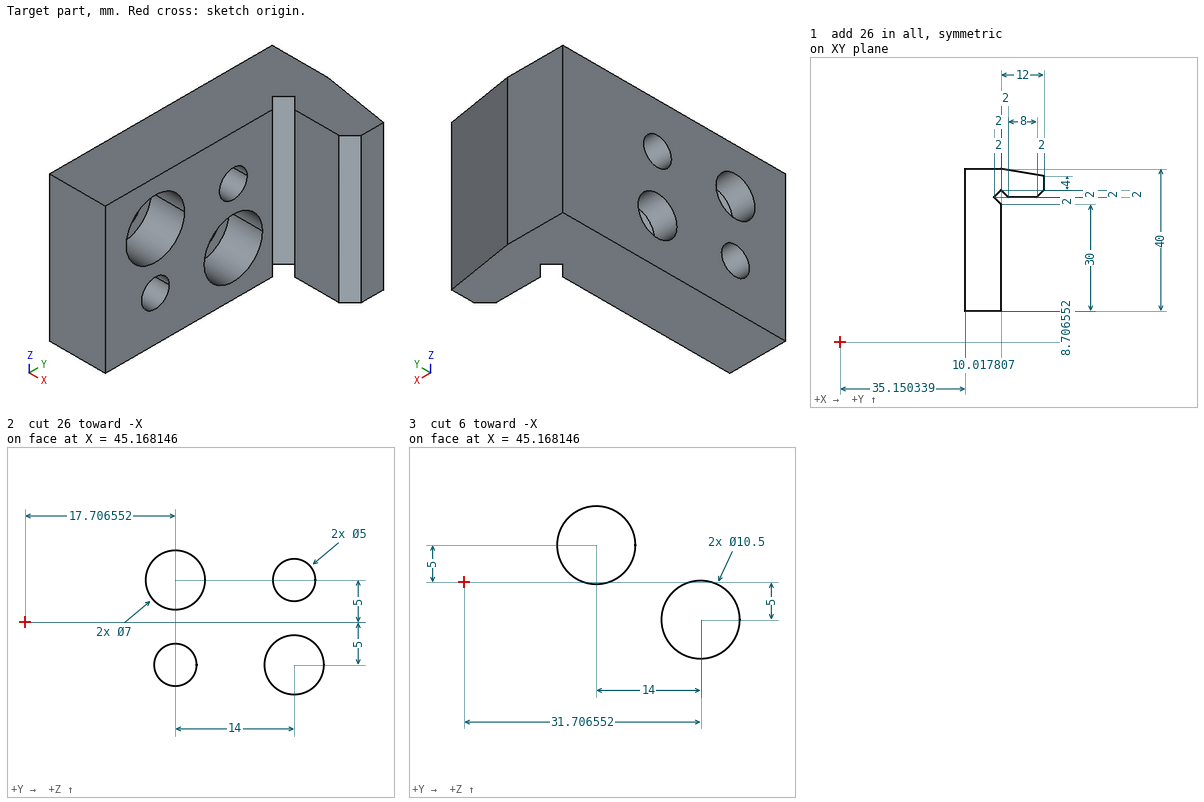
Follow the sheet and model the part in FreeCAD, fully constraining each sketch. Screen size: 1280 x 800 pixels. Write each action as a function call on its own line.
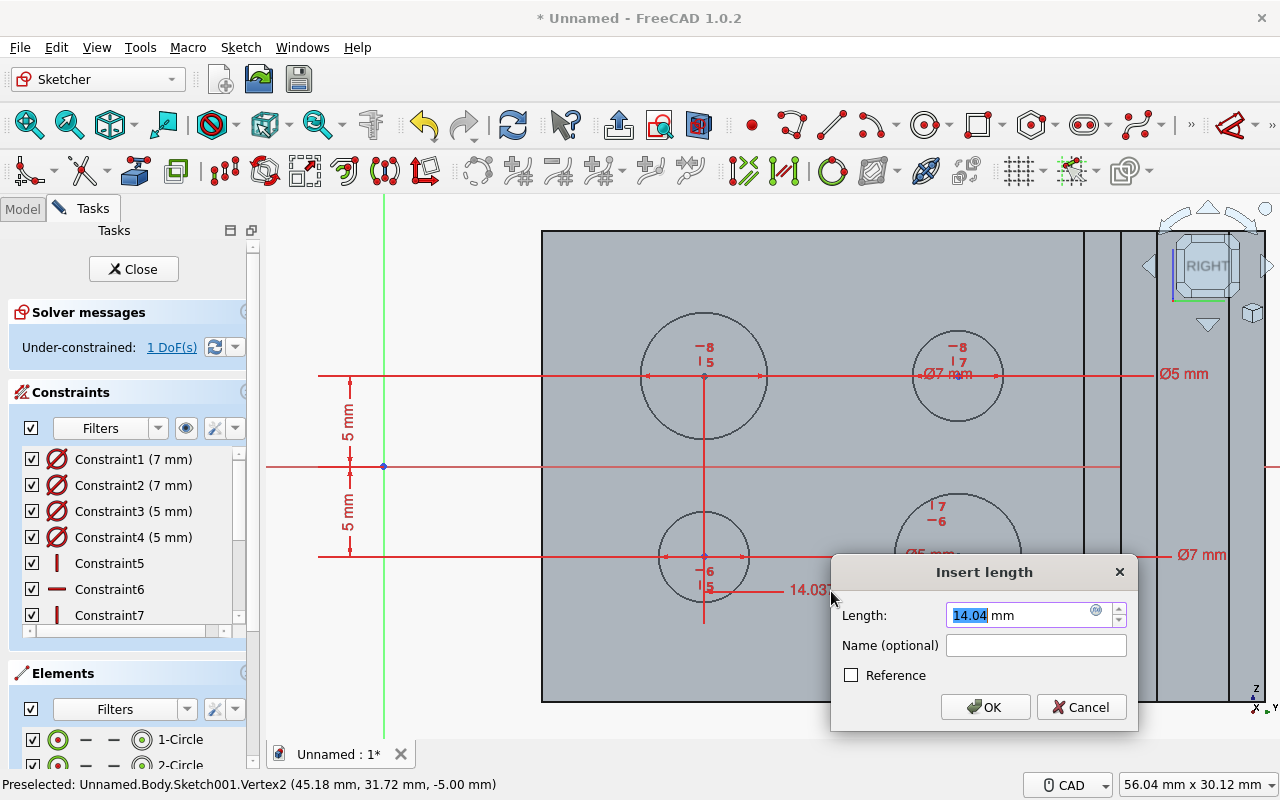
text(14)
key(Return)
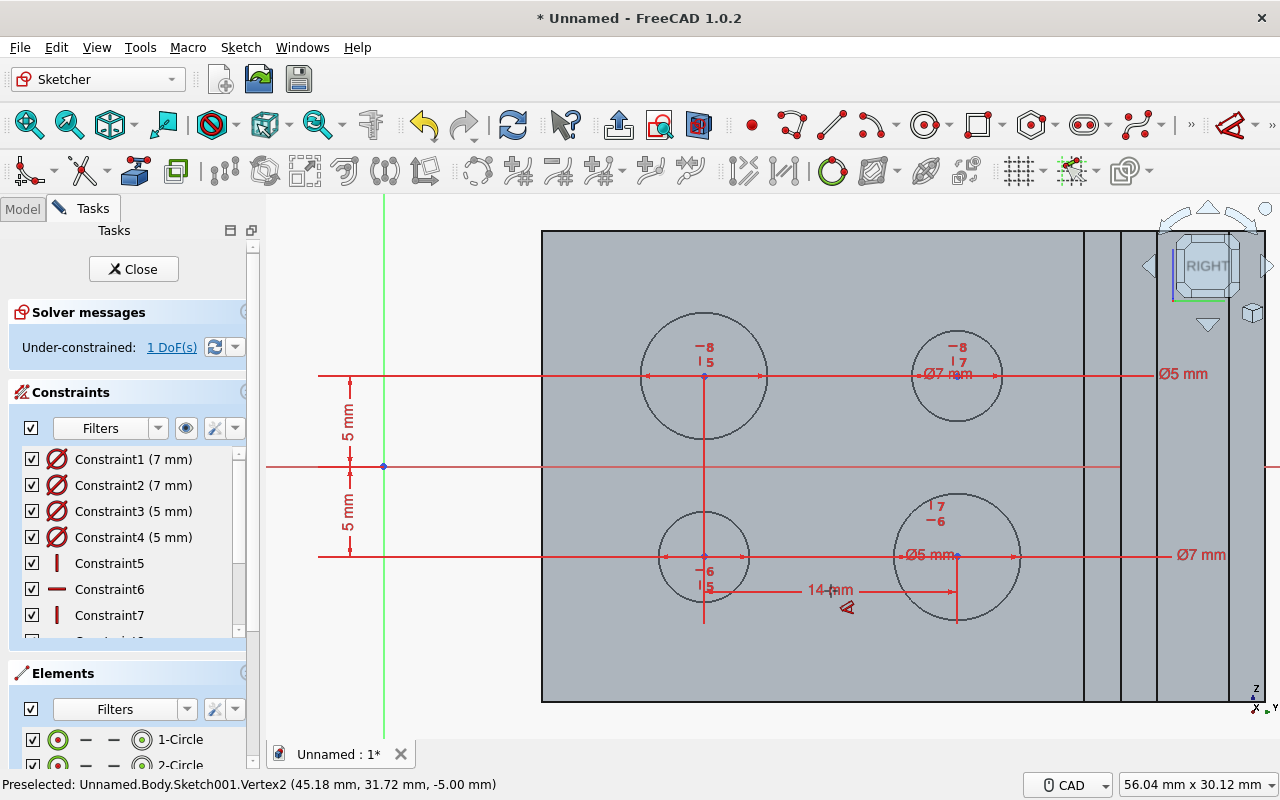
click(704, 376)
click(544, 342)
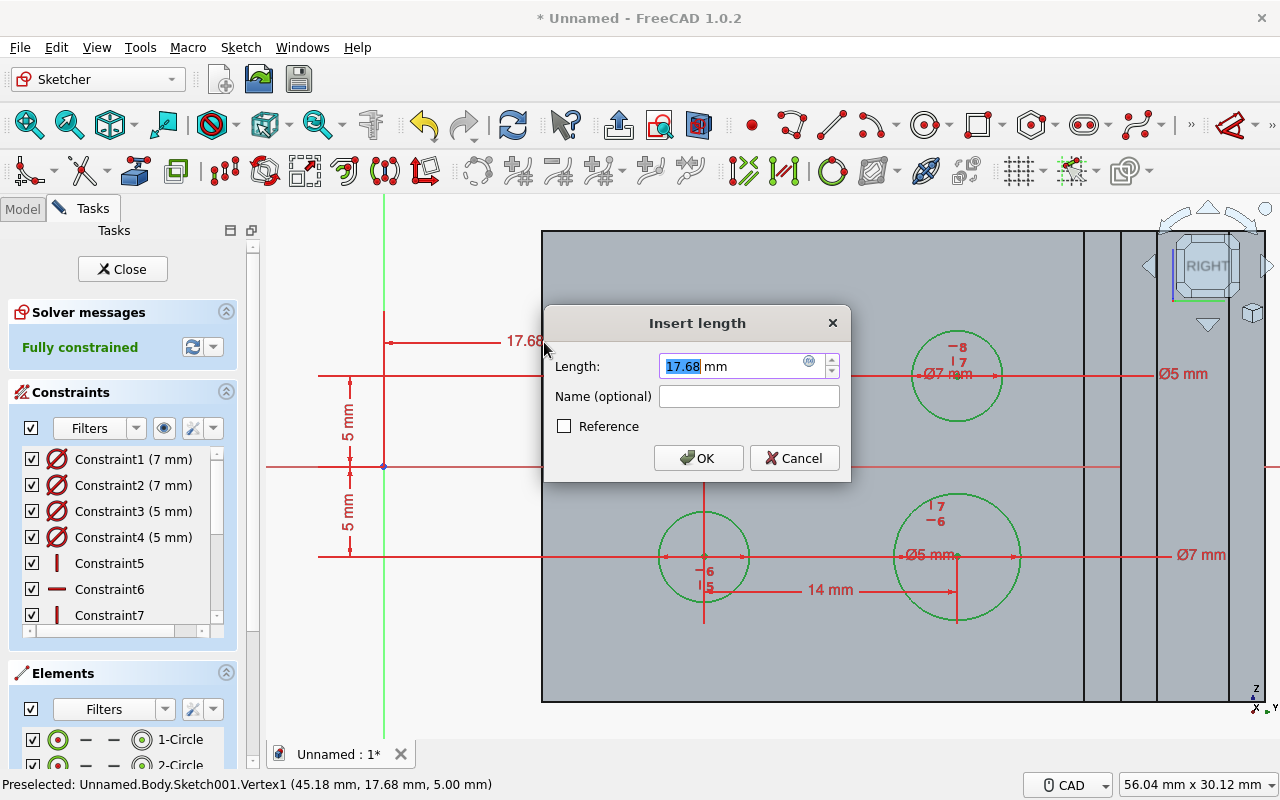
text(17.706552)
key(Return)
key(Escape)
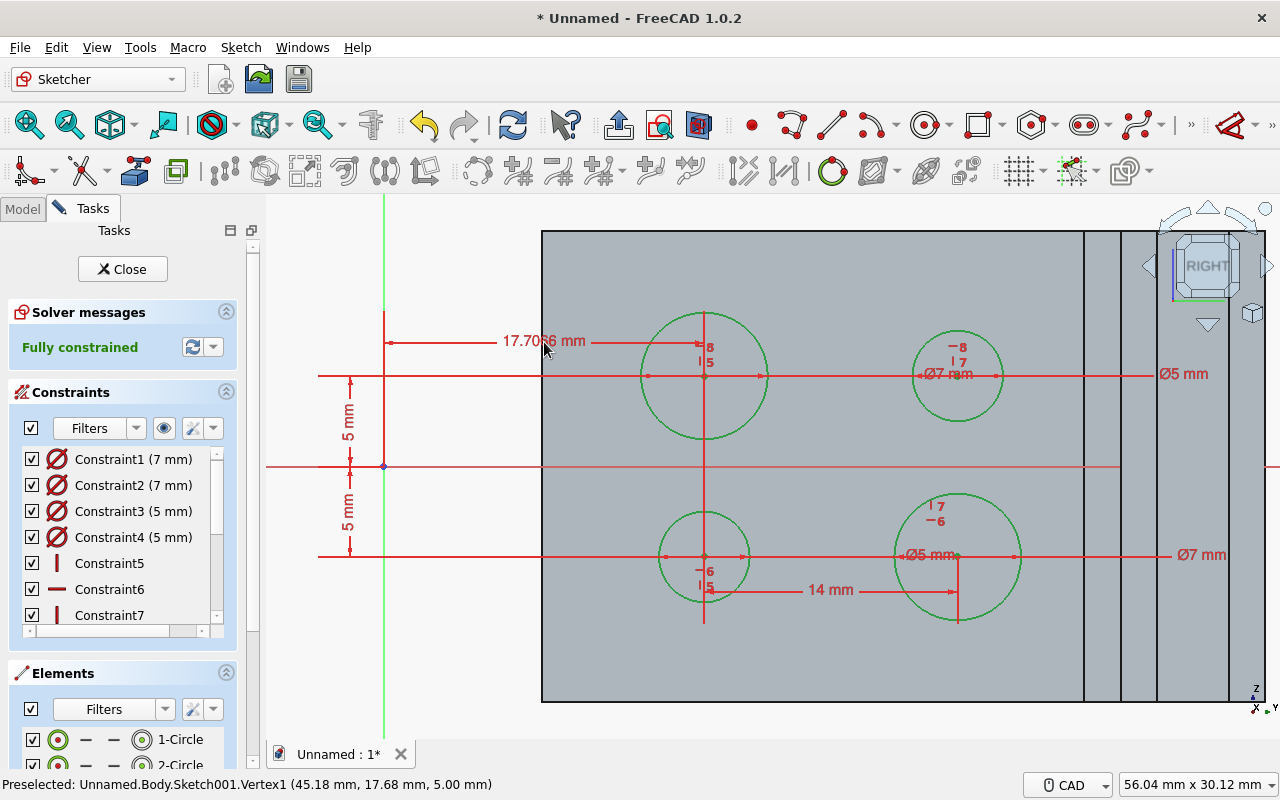
click(123, 269)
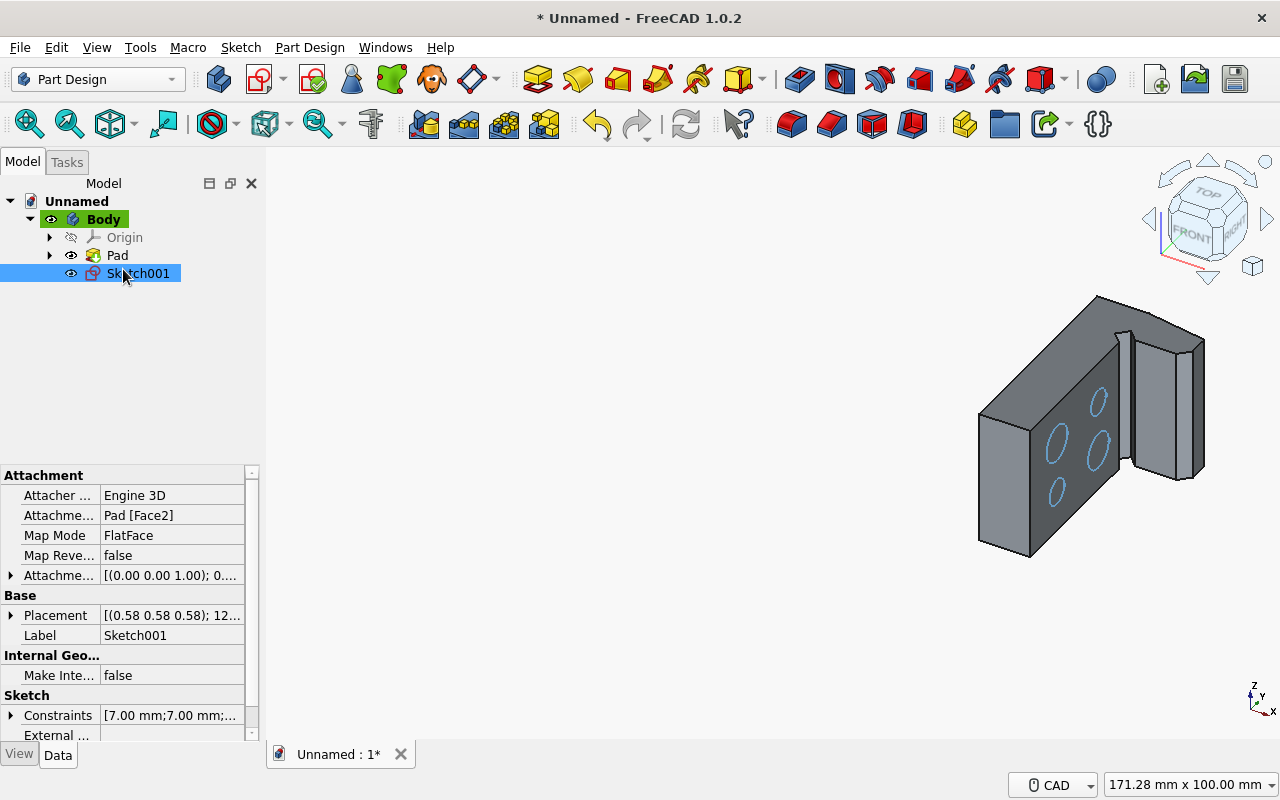
click(800, 80)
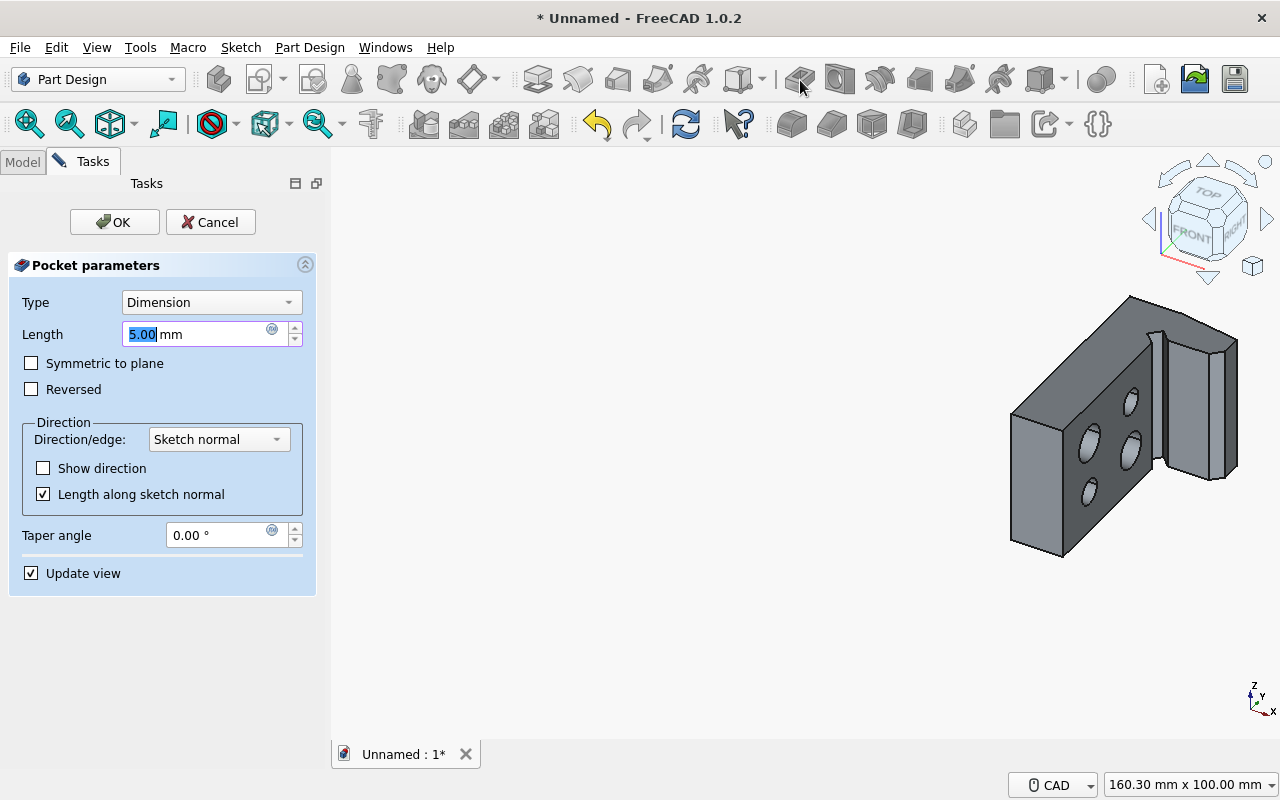
text(26)
key(Tab)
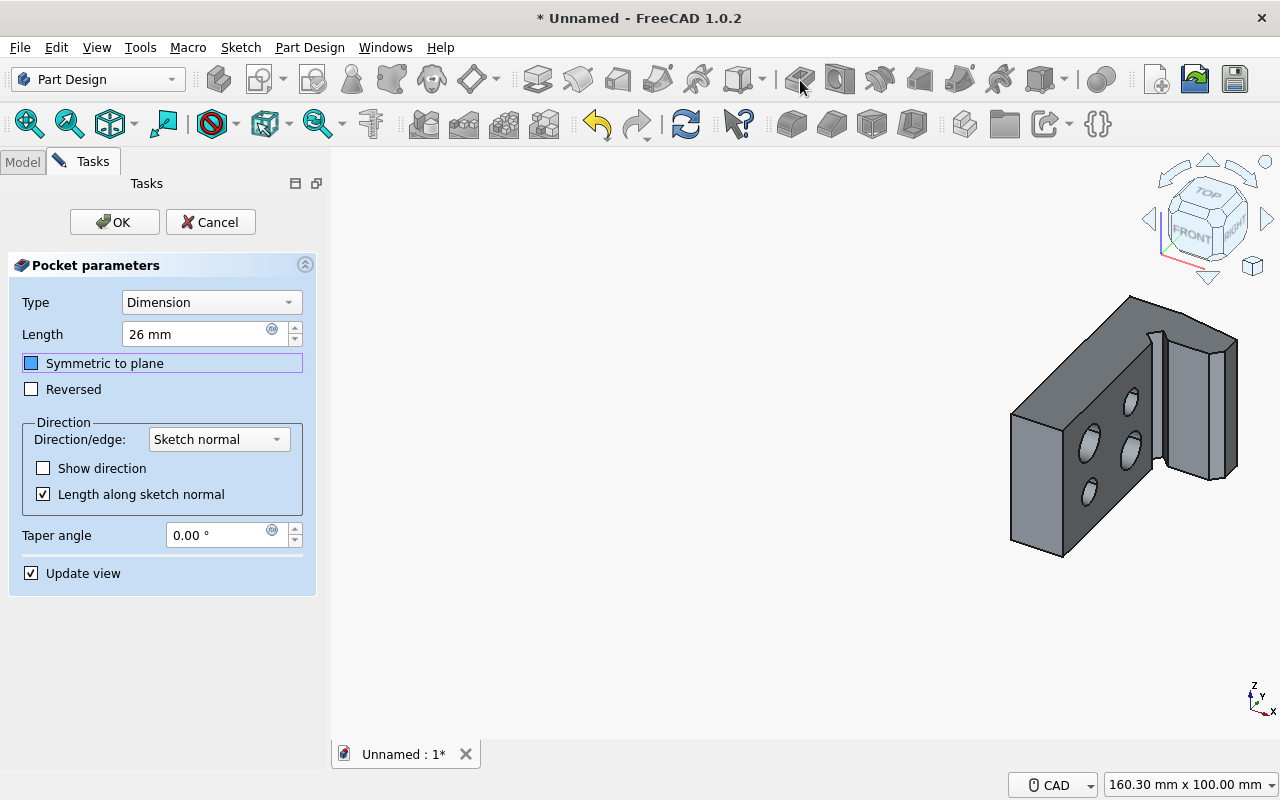
click(115, 222)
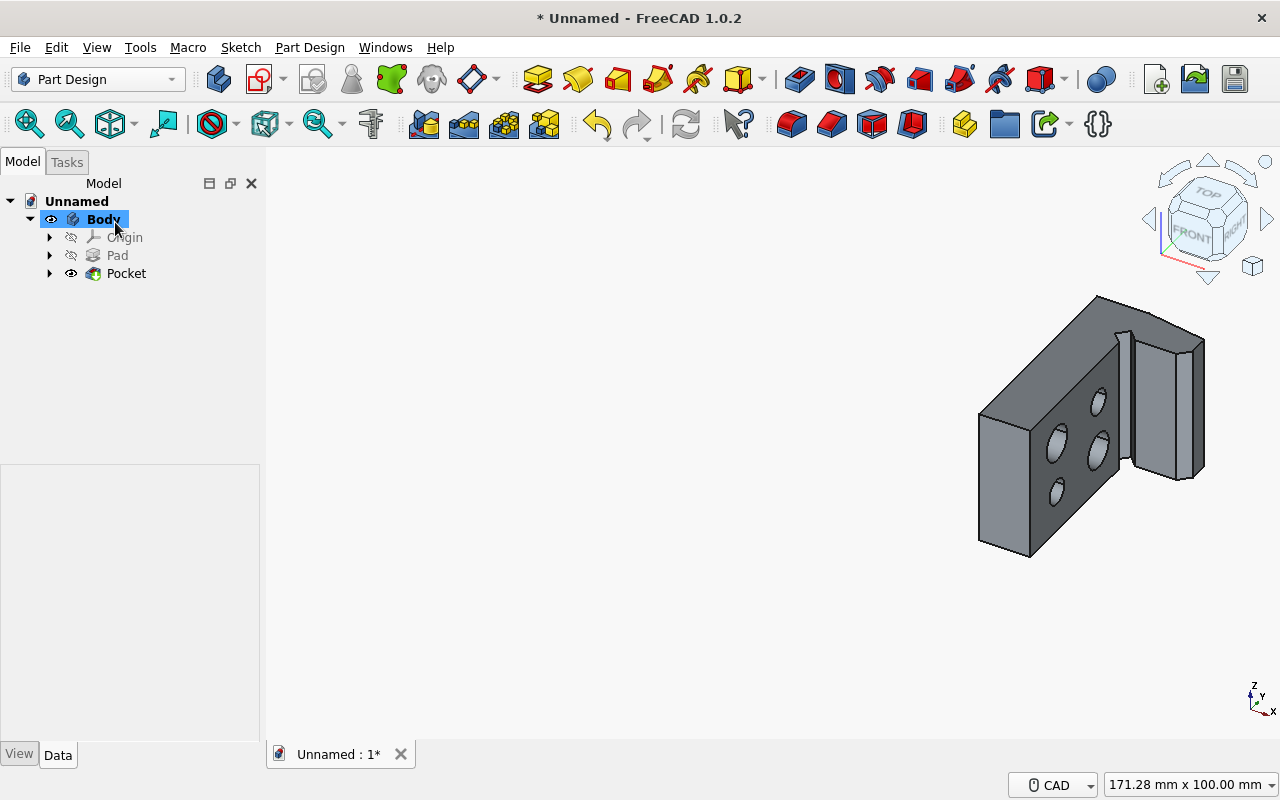
click(1075, 449)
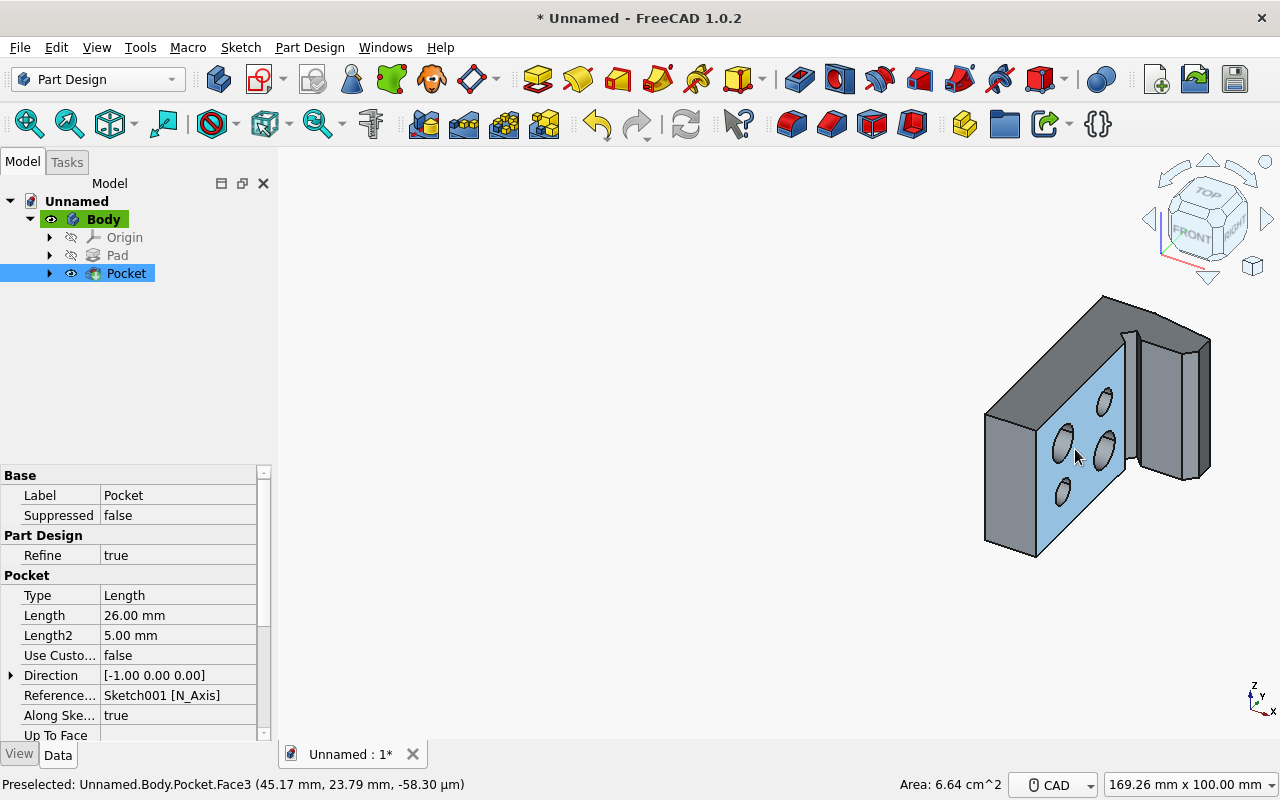
click(260, 80)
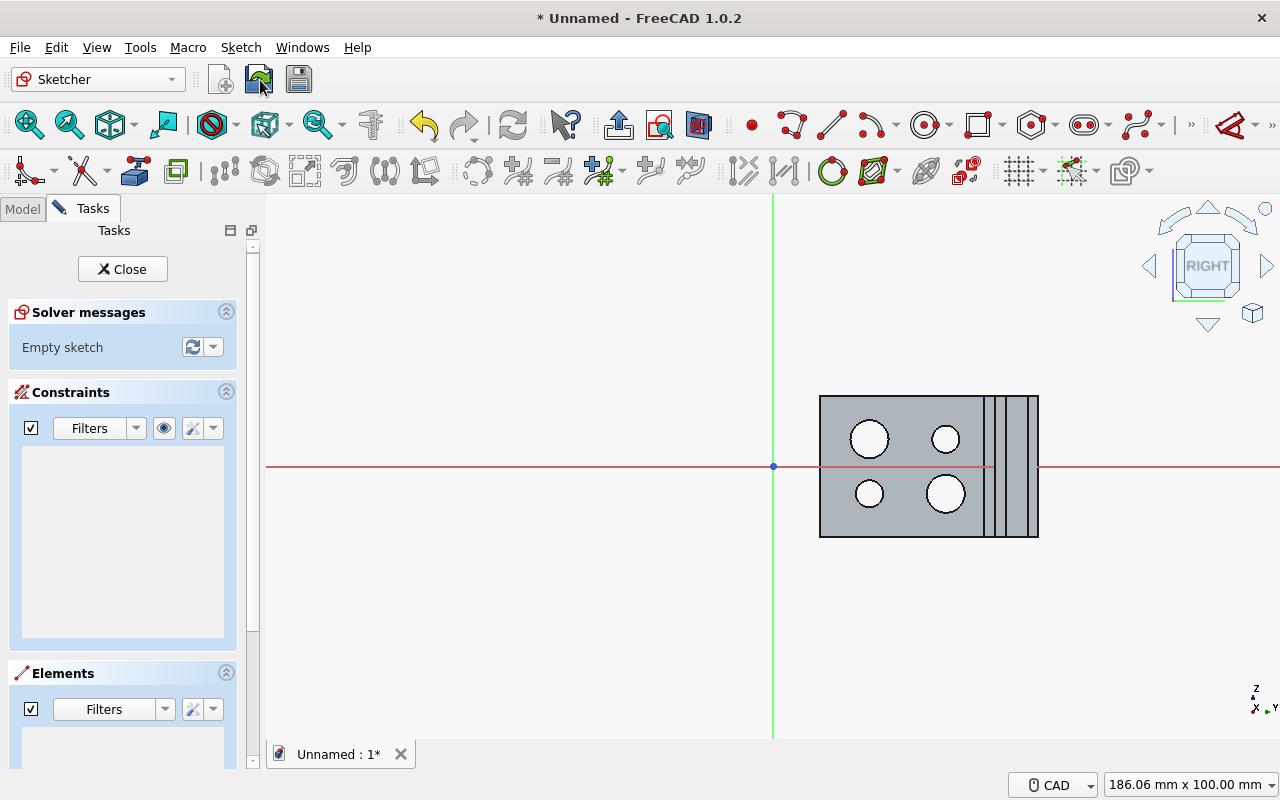
key(q)
key(s)